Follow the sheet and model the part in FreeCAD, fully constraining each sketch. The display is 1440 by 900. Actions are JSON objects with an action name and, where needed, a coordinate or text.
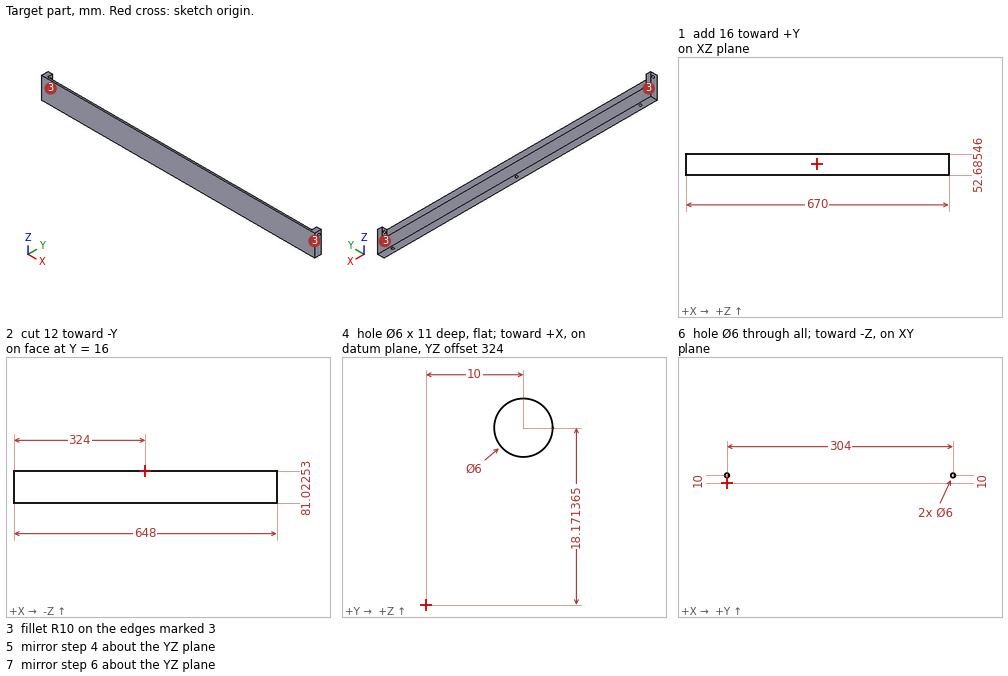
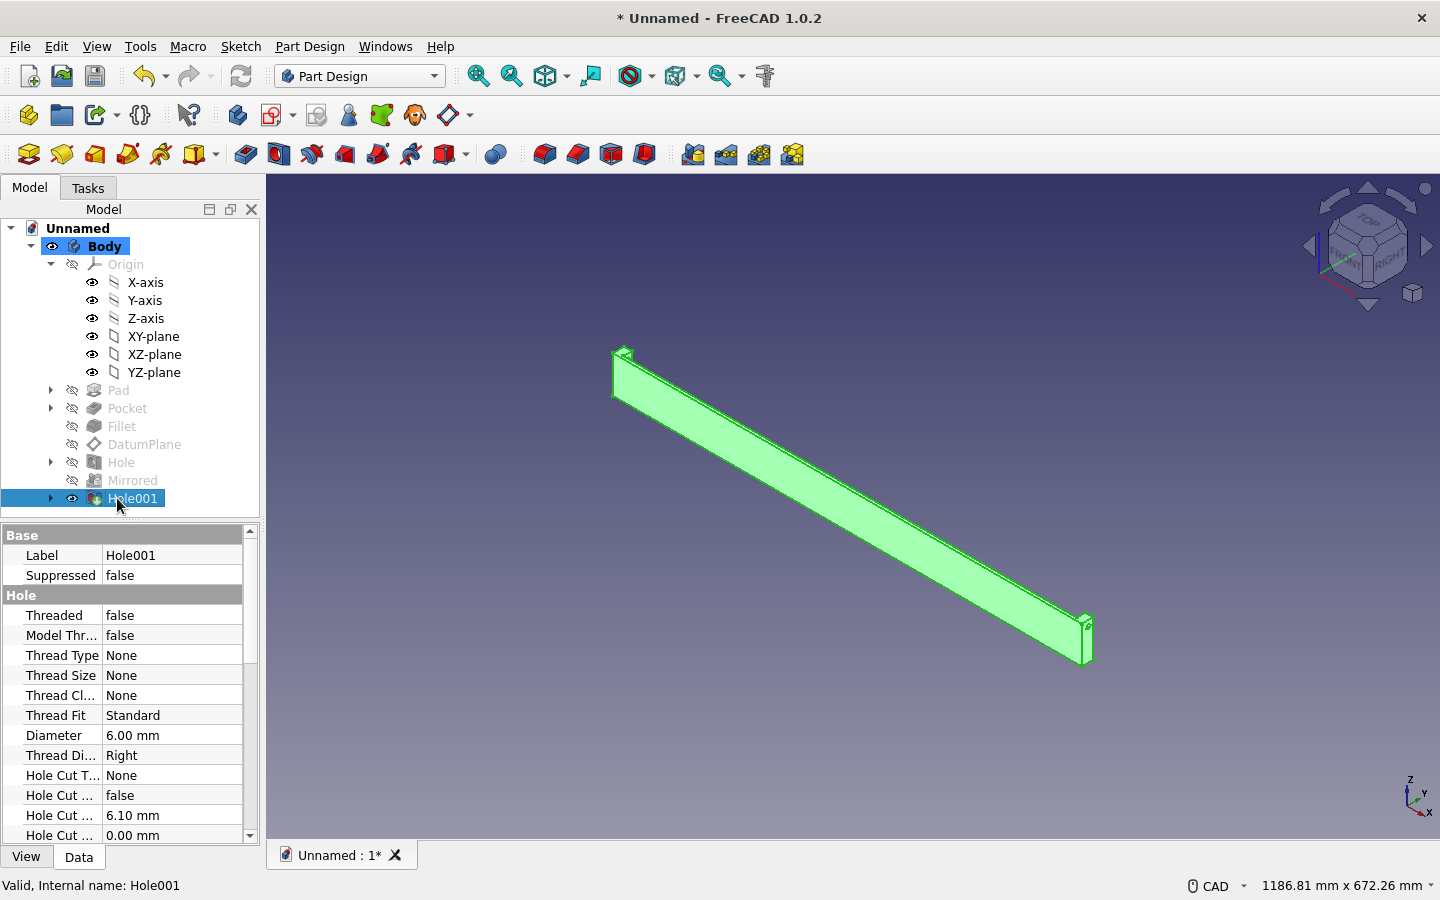
{"action": "left_click", "coordinate": [693, 154]}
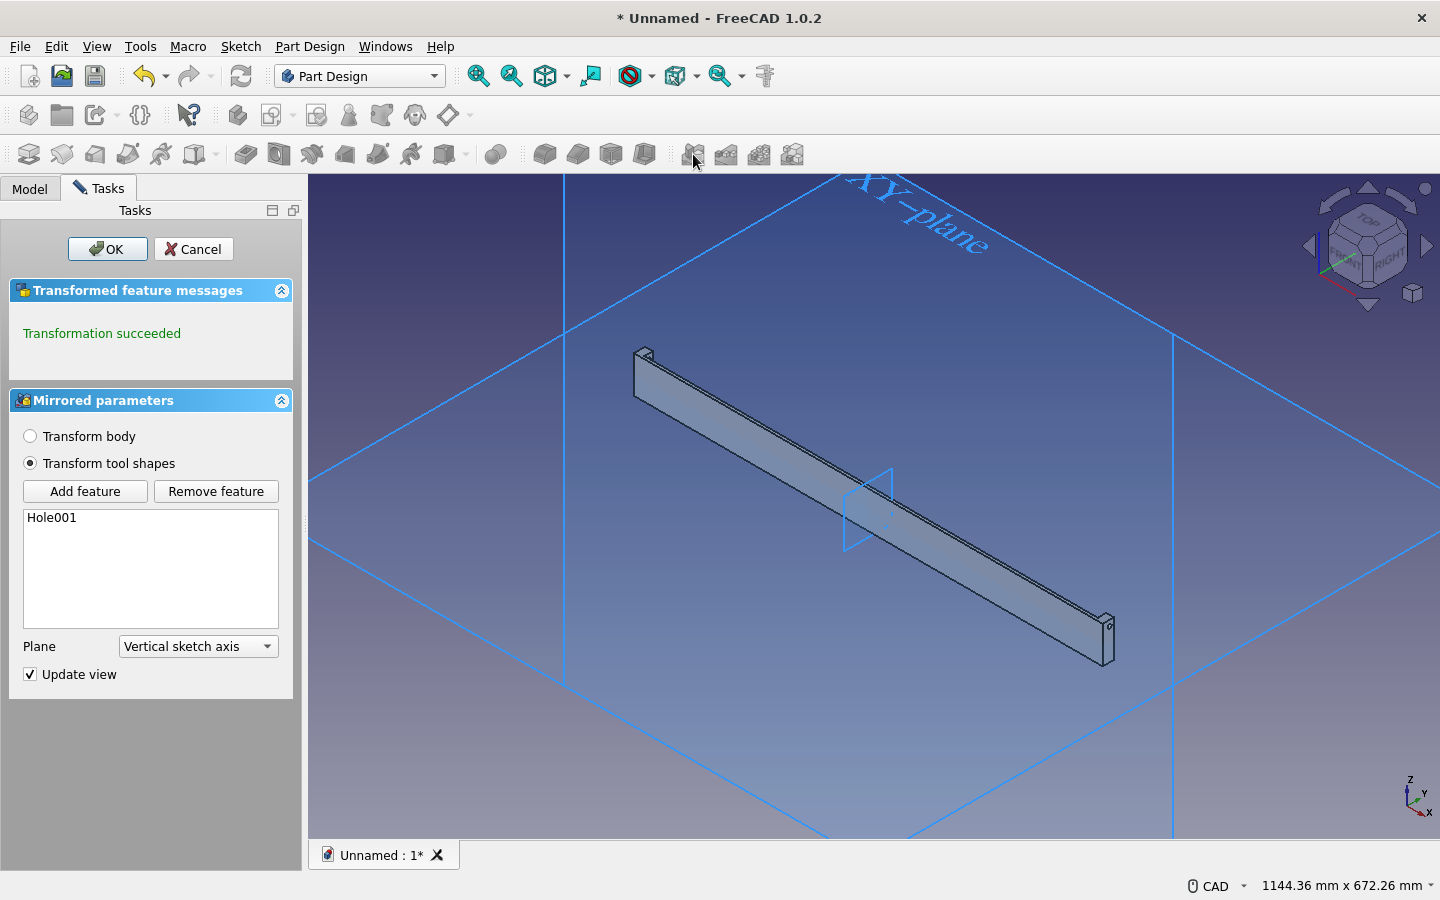
{"action": "left_click", "coordinate": [199, 646]}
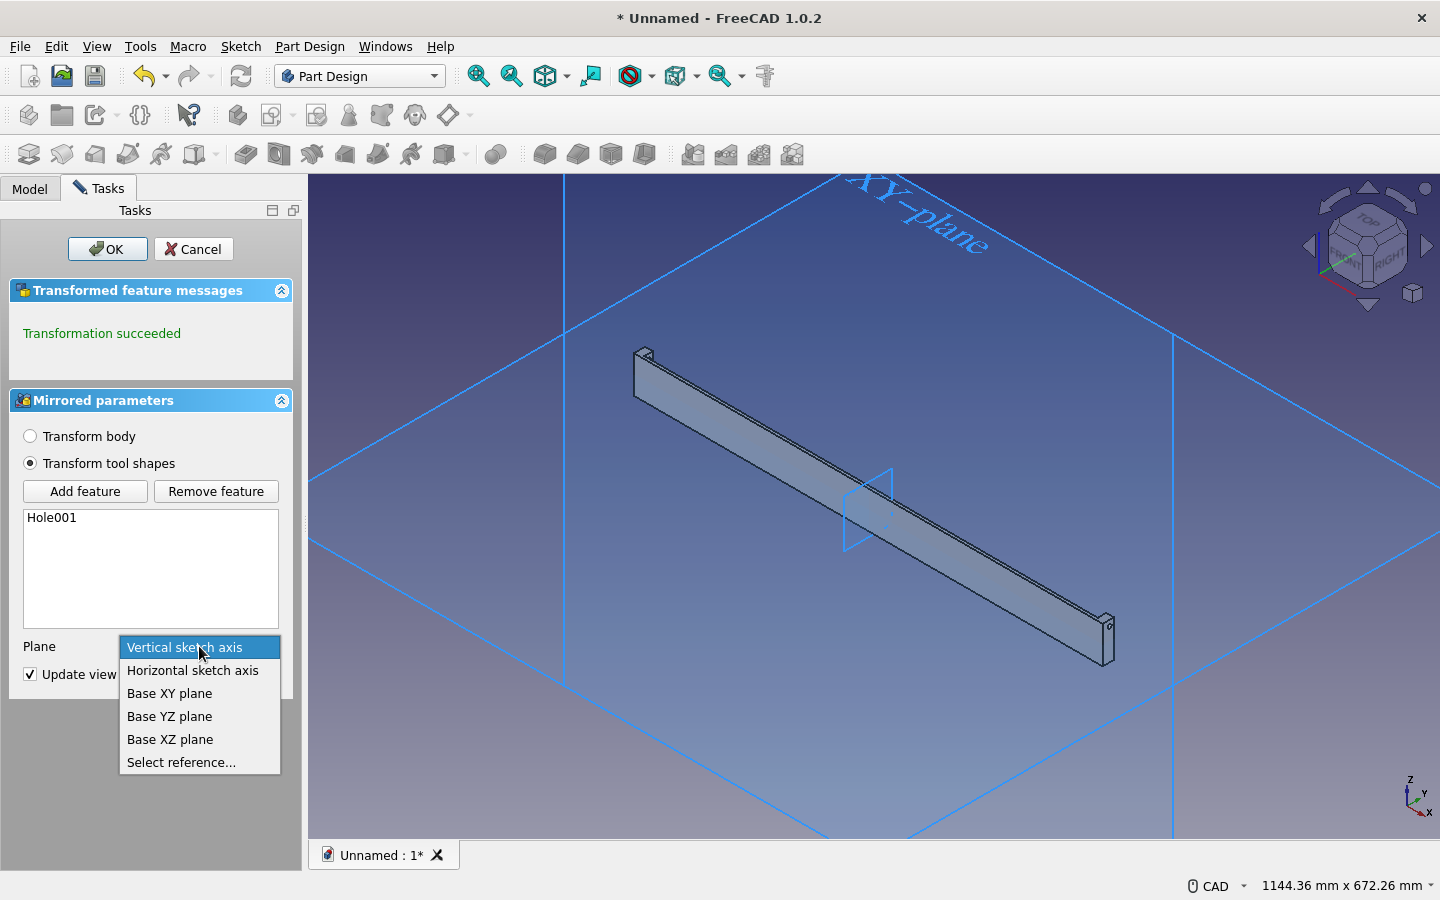
{"action": "left_click", "coordinate": [198, 716]}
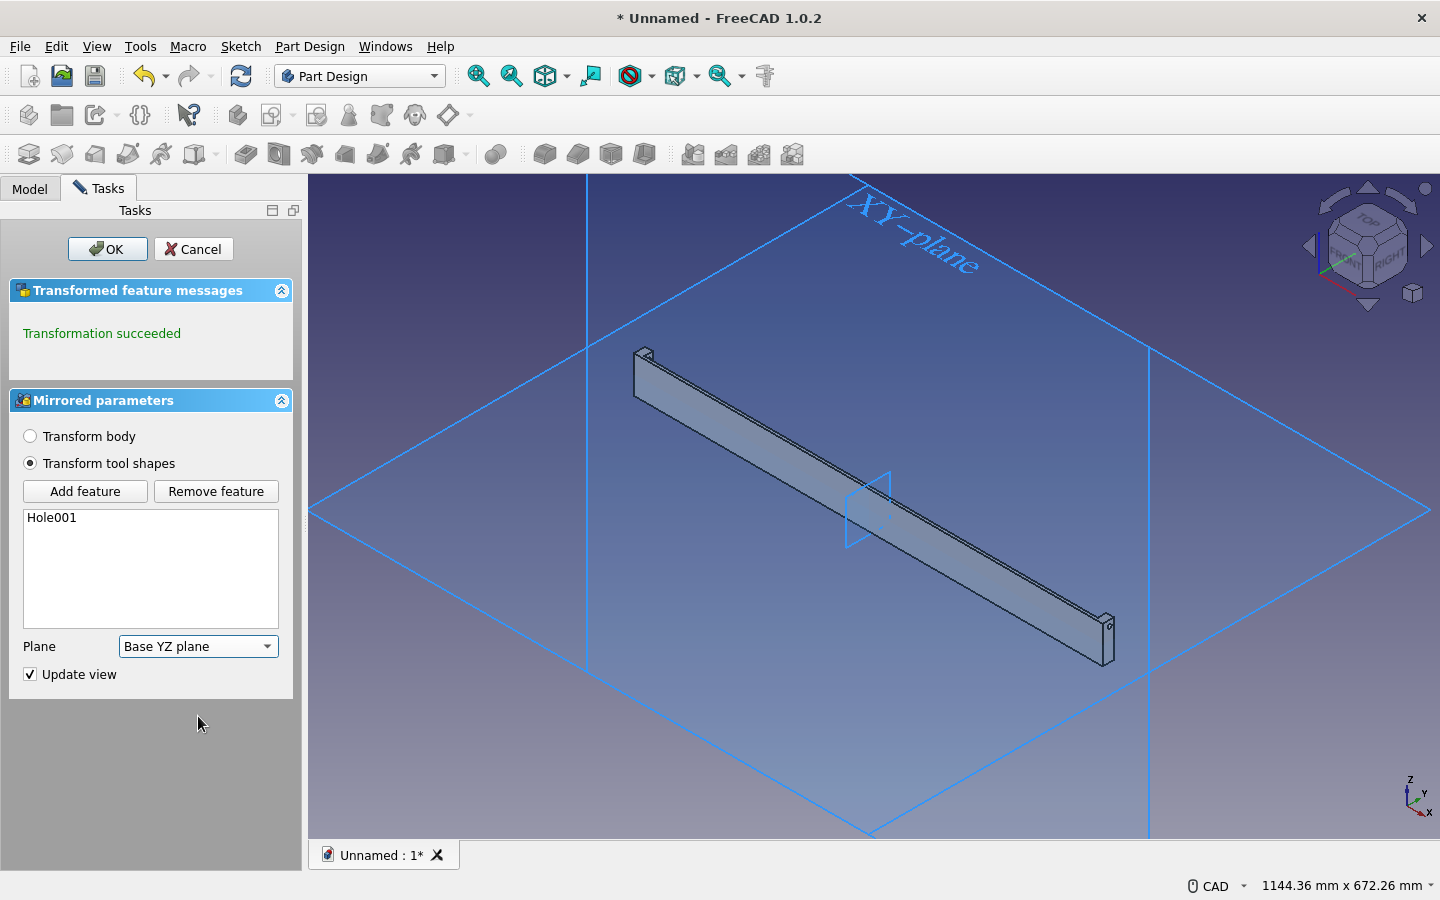
{"action": "left_click", "coordinate": [108, 249]}